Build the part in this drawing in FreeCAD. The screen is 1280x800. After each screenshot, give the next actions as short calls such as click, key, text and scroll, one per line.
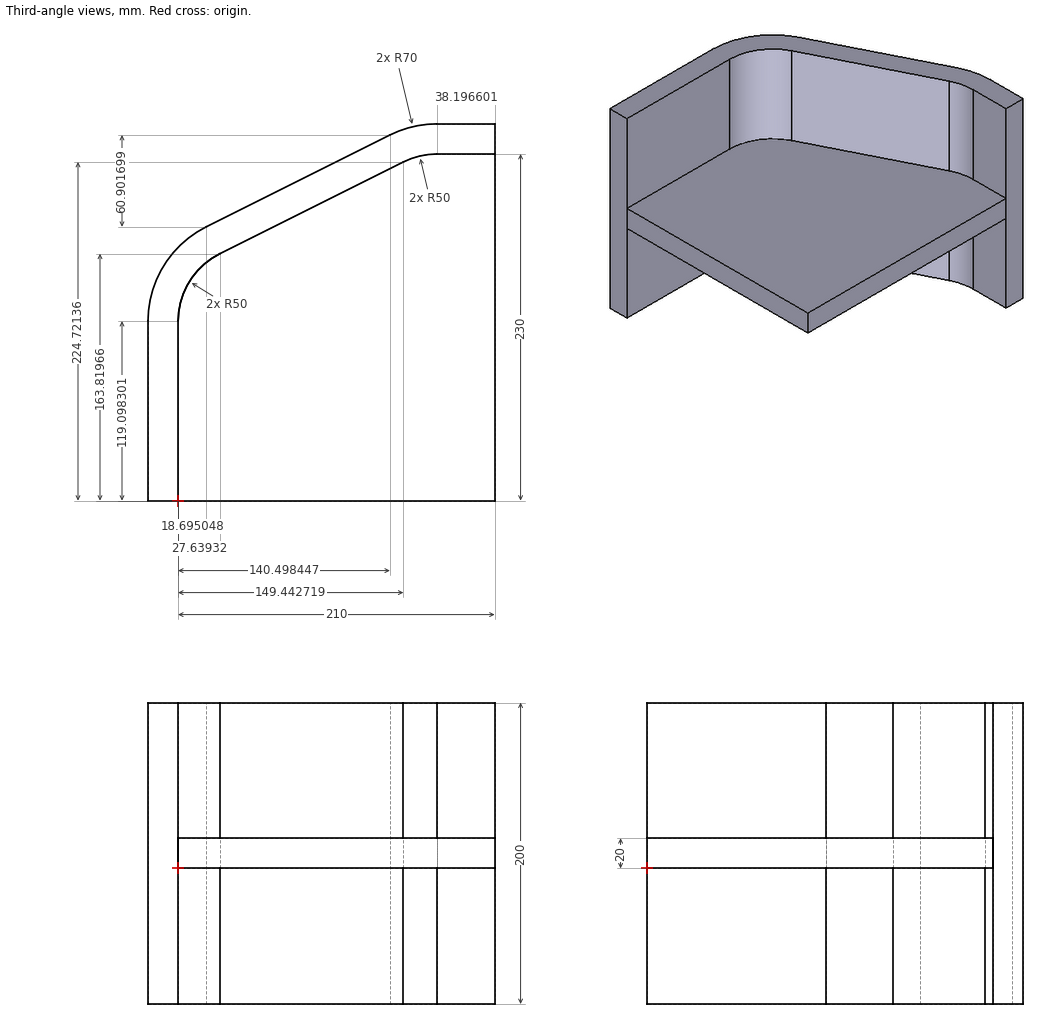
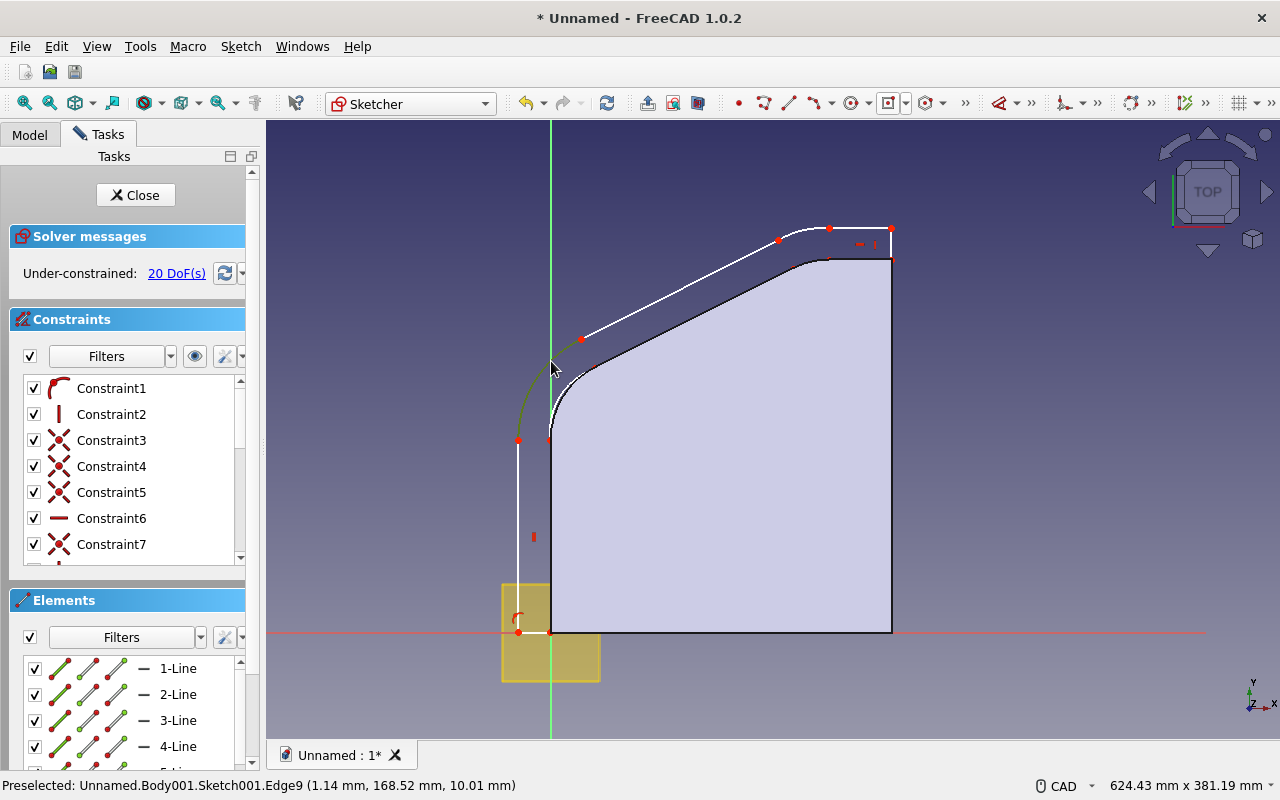
click(572, 382)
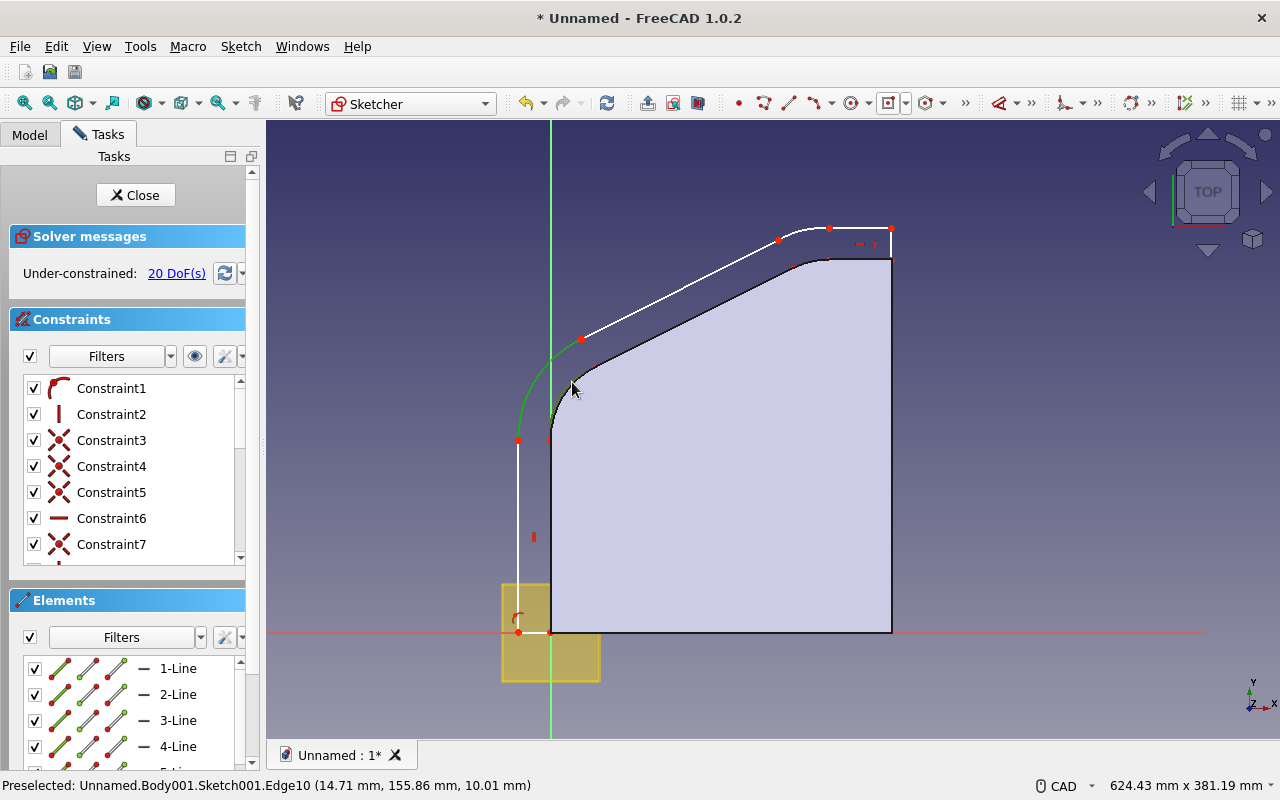
key(c)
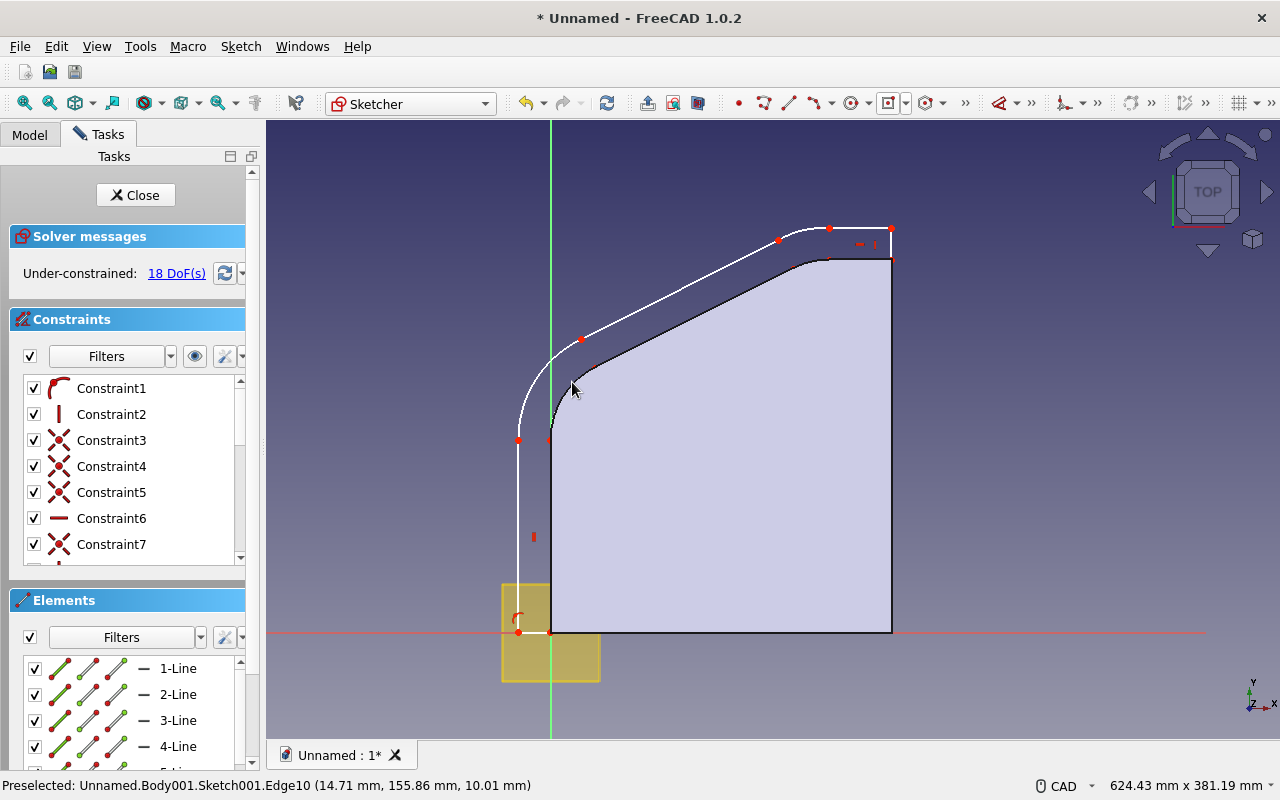
click(818, 260)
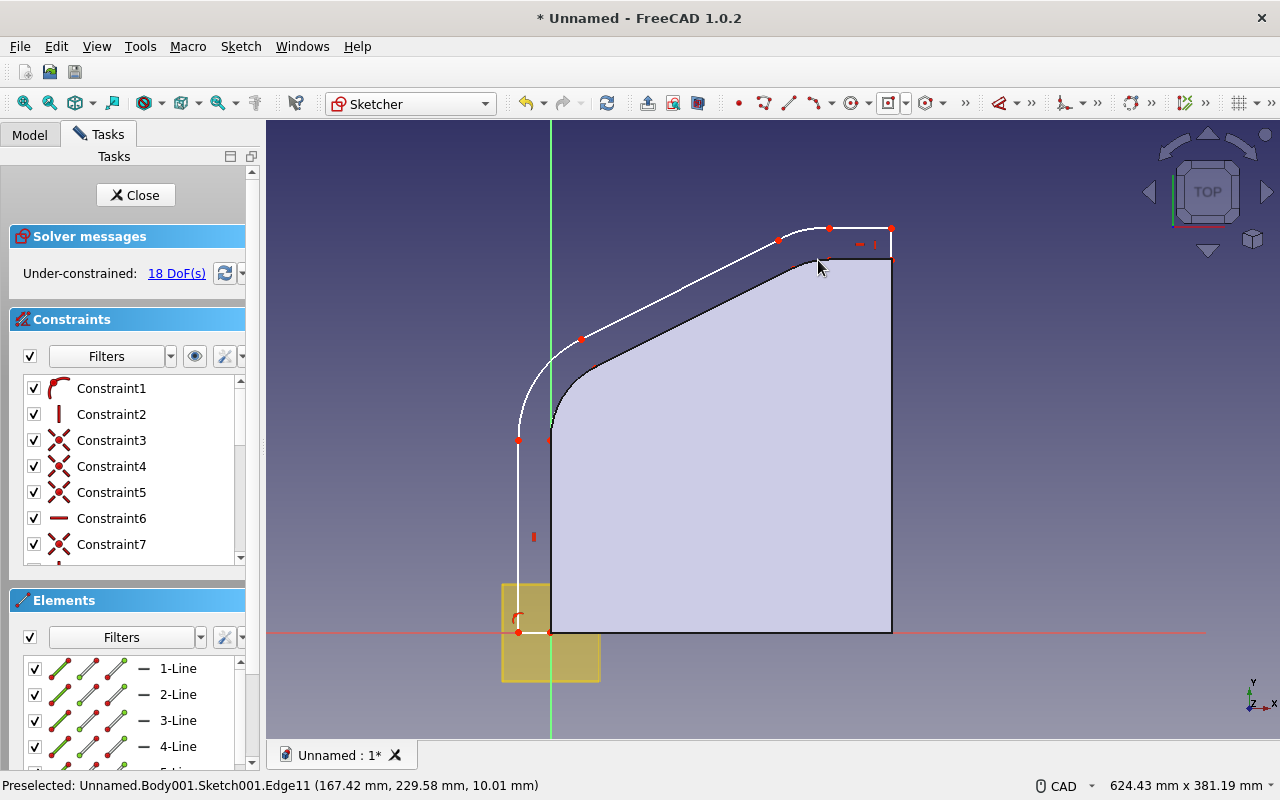
click(813, 229)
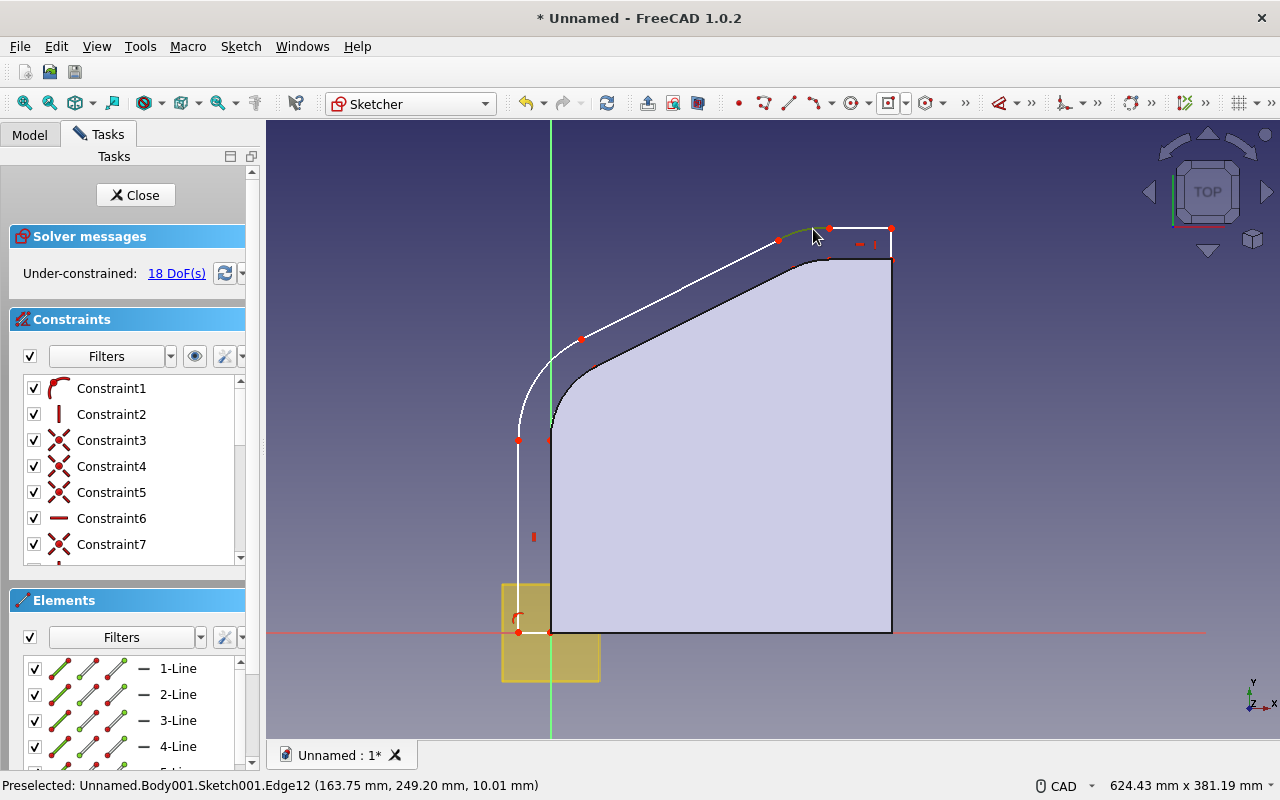
key(c)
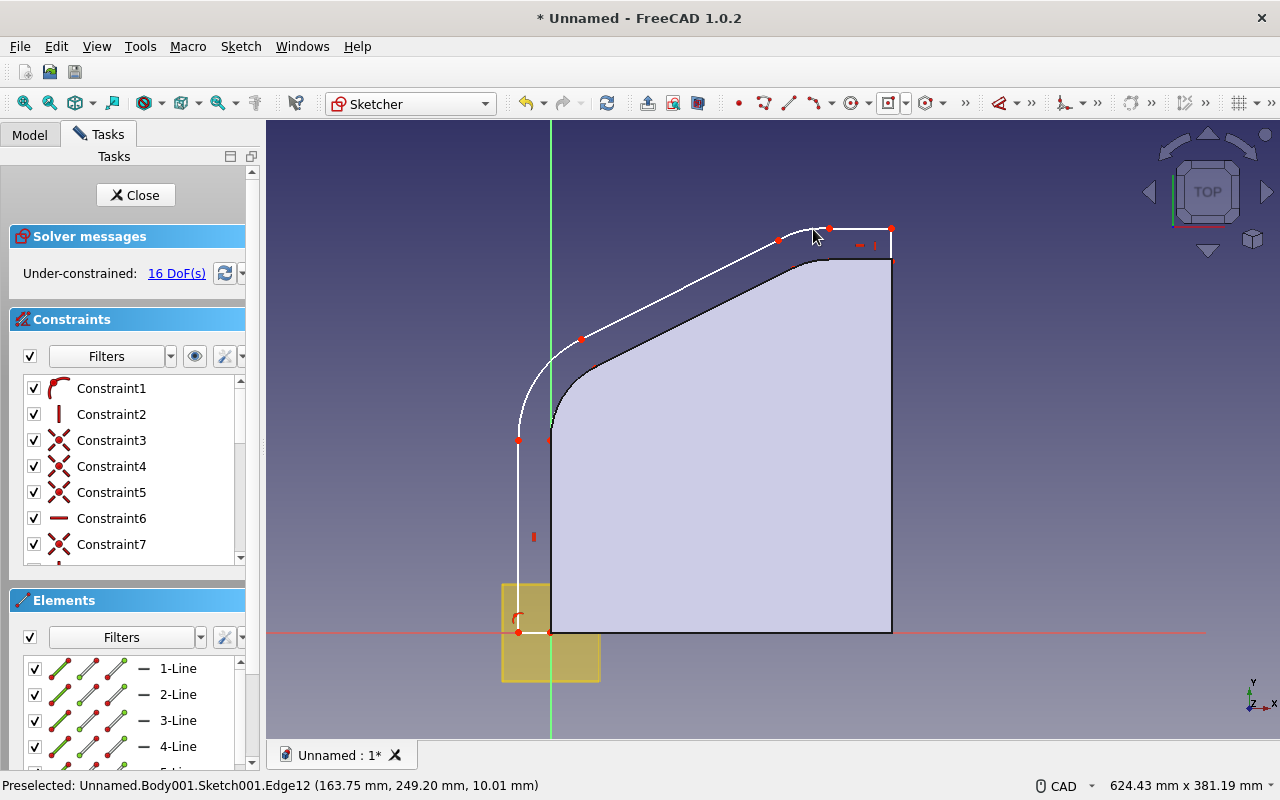
click(574, 384)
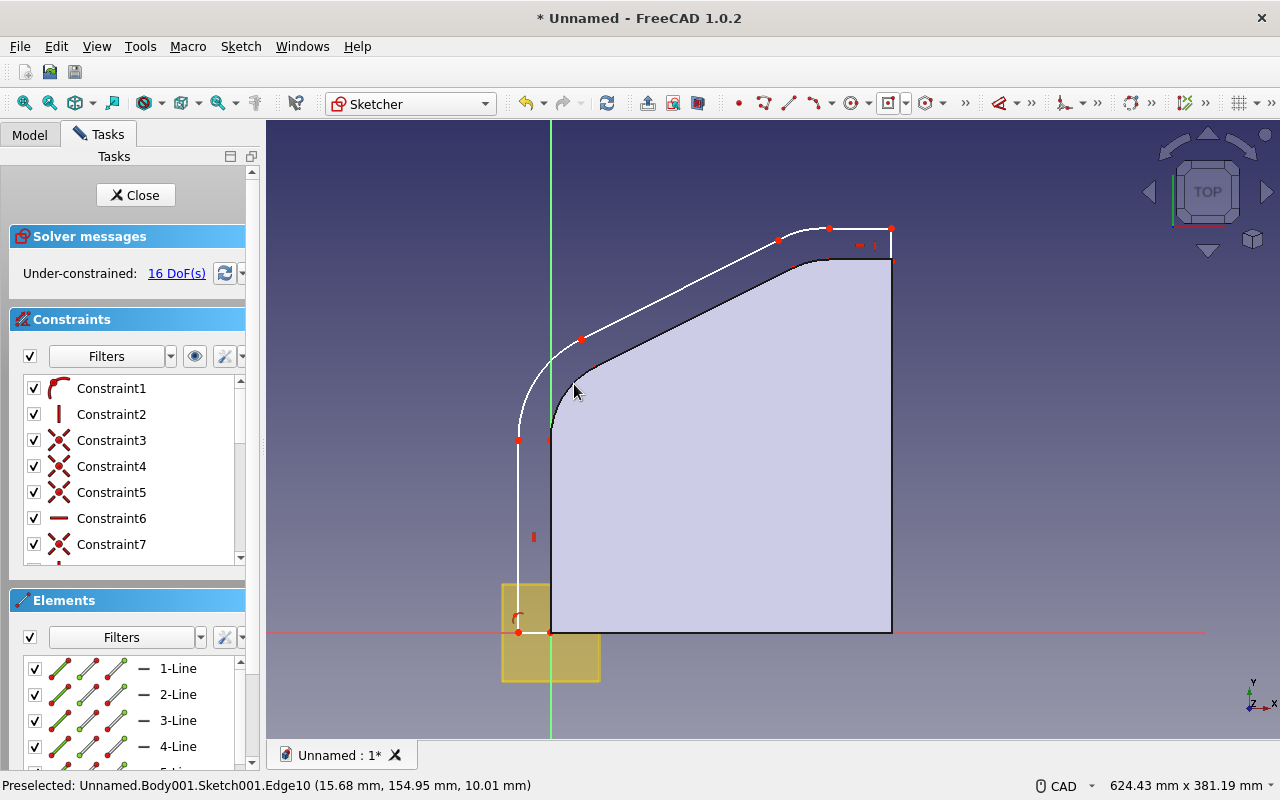
scroll(818, 261, up, 2)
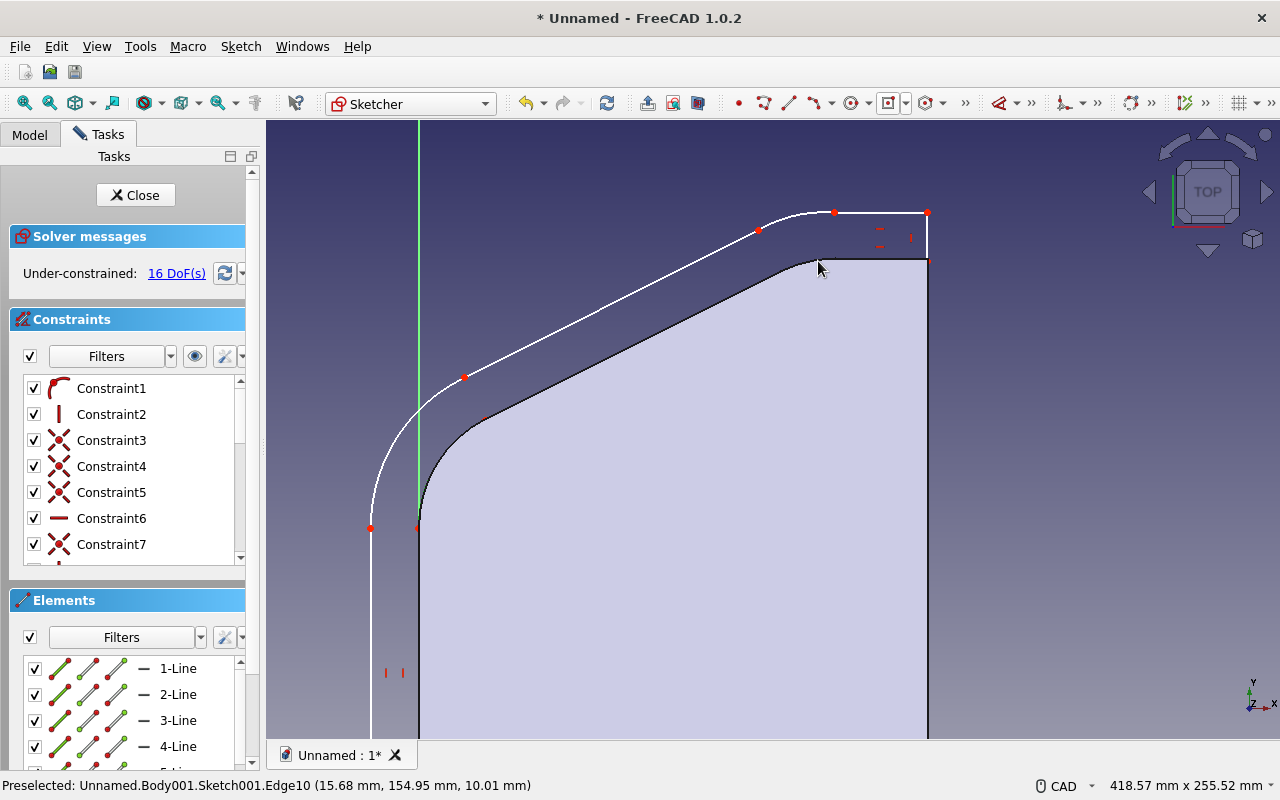
click(818, 261)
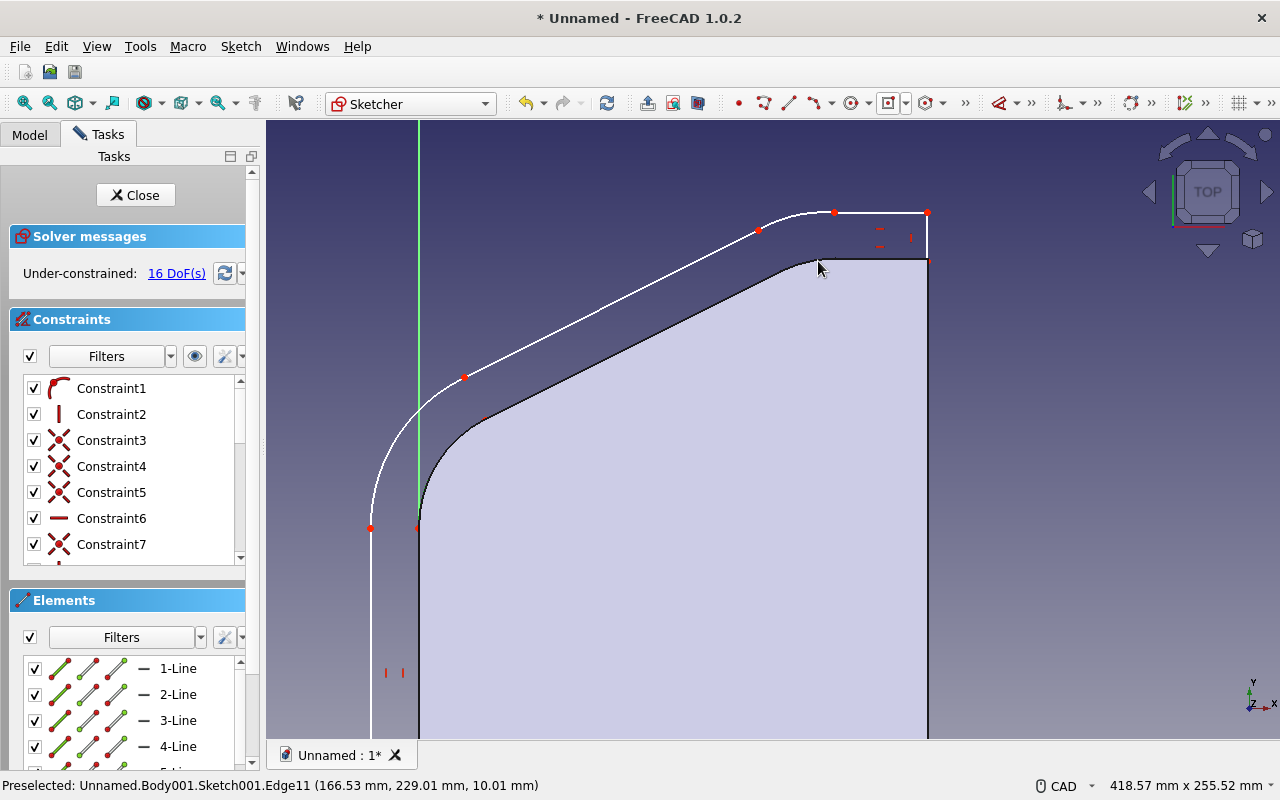
key(e)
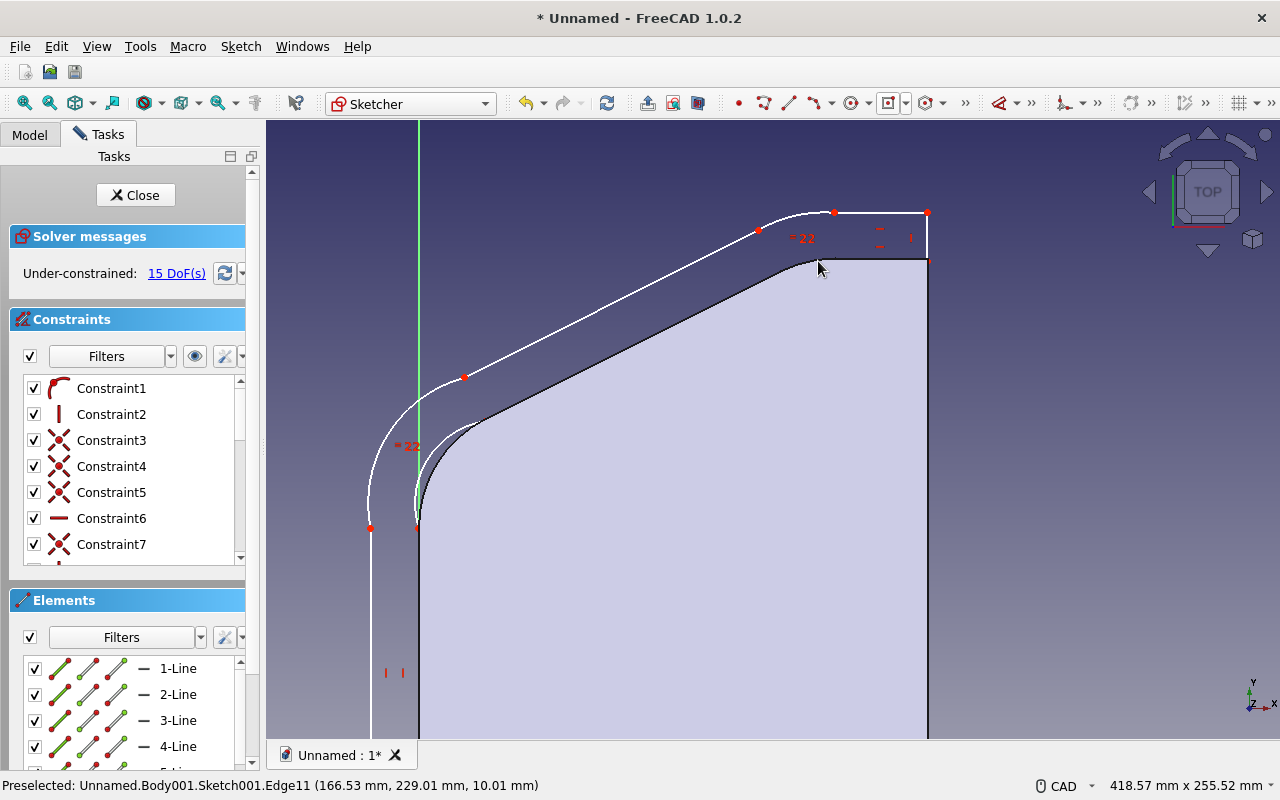
click(373, 470)